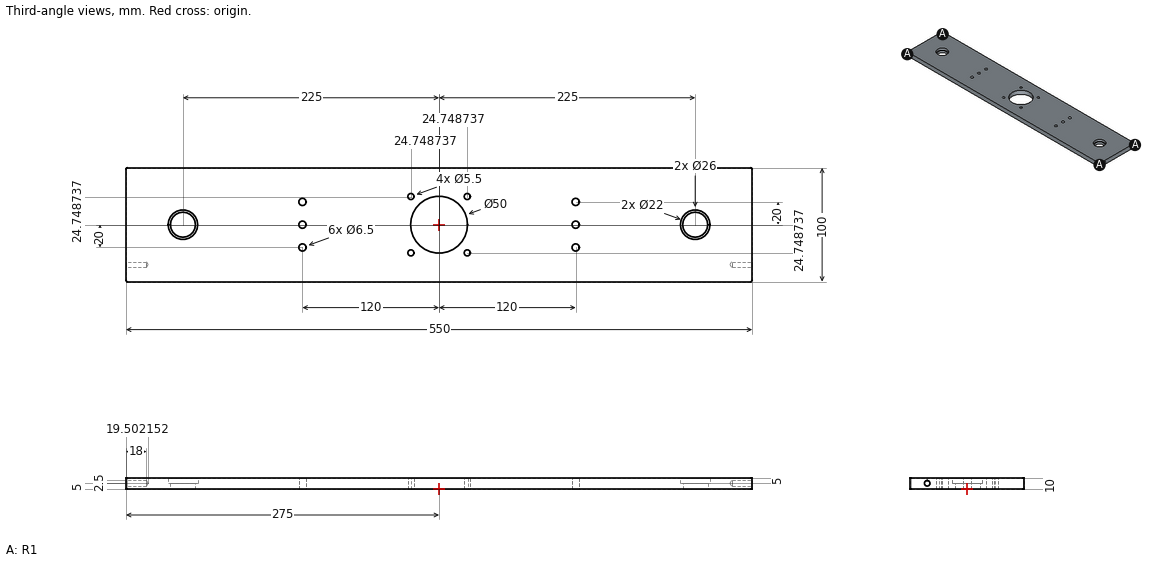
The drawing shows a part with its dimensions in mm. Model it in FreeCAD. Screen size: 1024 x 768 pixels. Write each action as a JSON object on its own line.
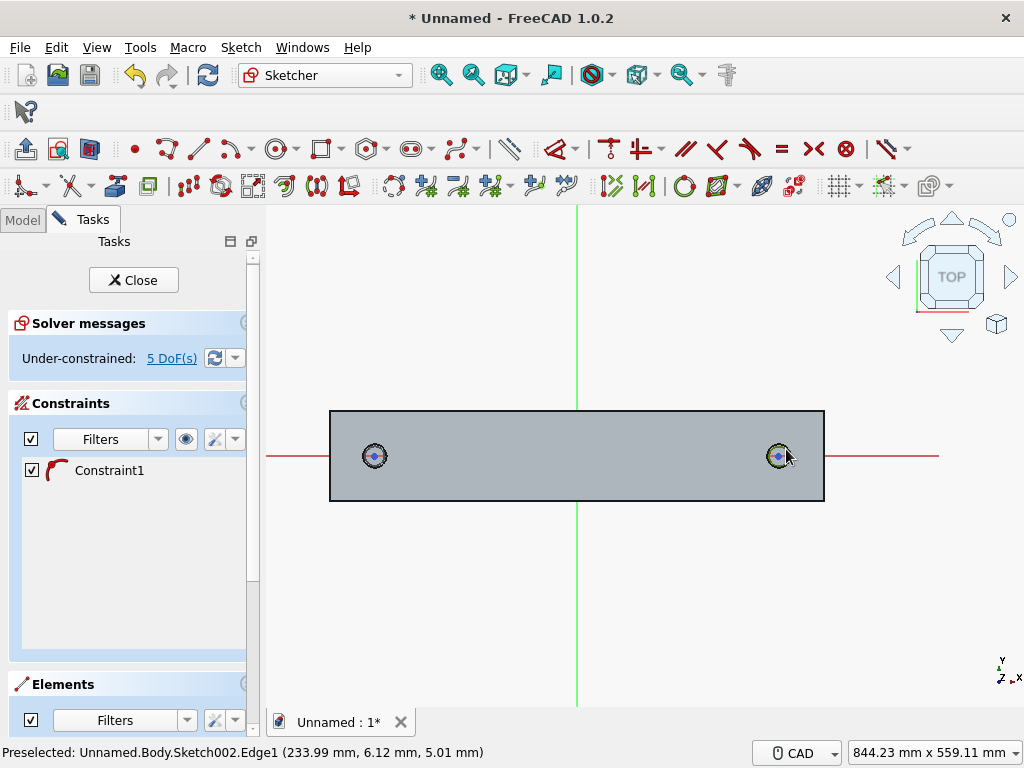
{"action": "scroll", "coordinate": [382, 449], "scroll_direction": "up", "scroll_amount": 4}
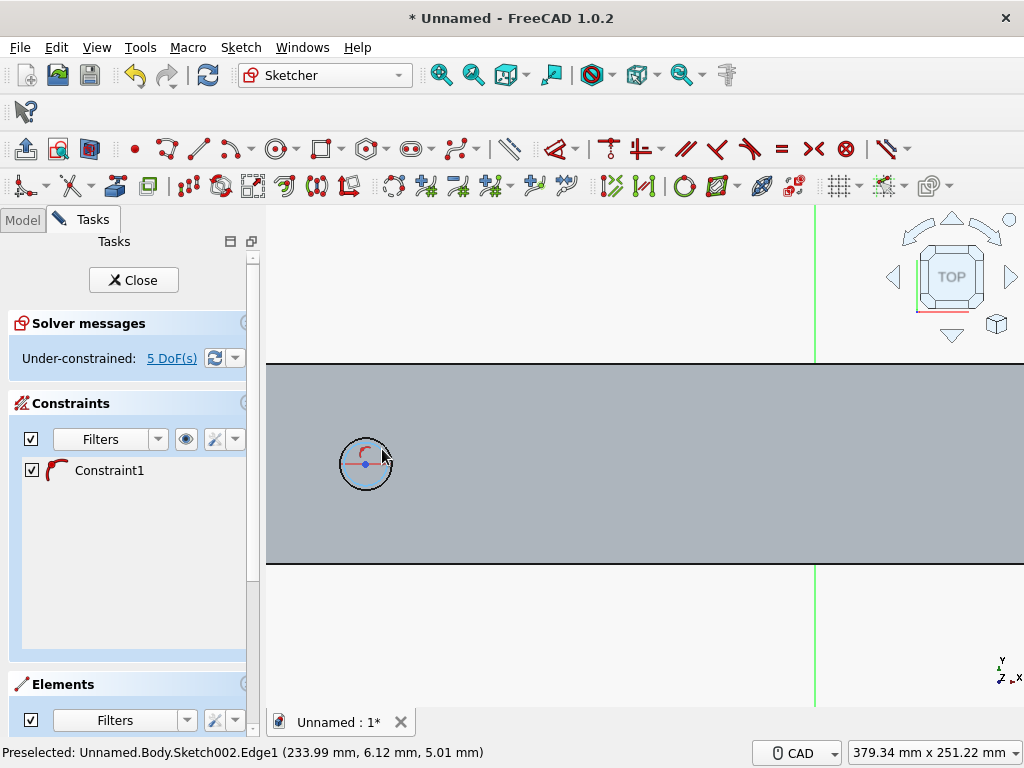
{"action": "left_click", "coordinate": [381, 449]}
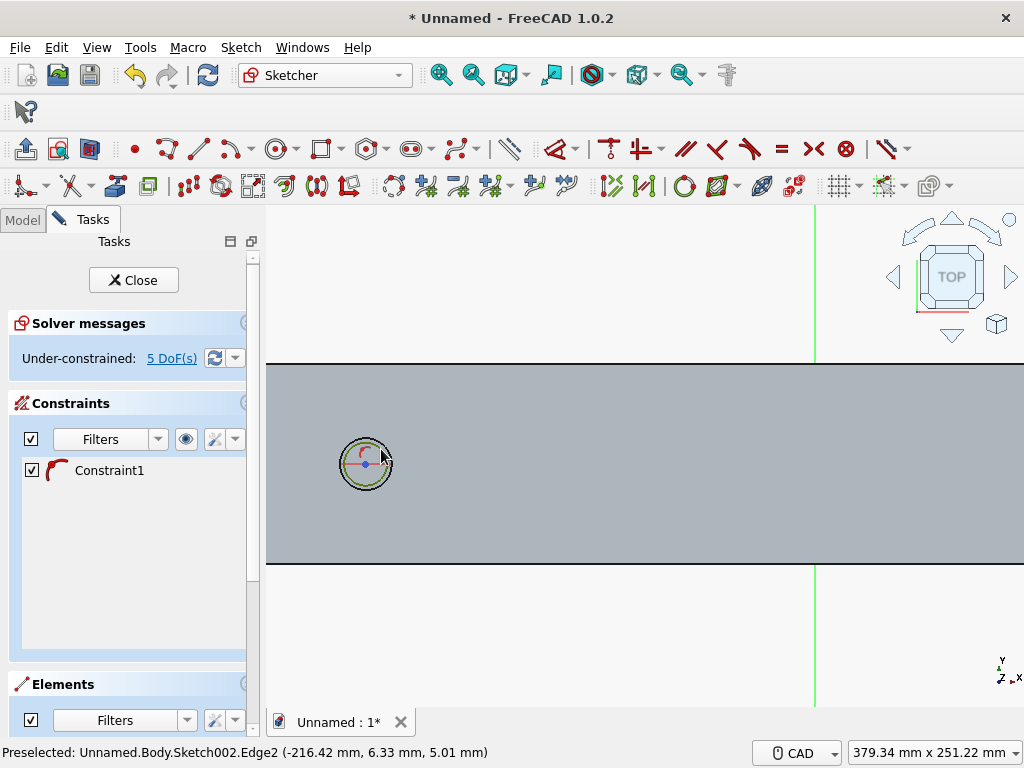
{"action": "left_click", "coordinate": [782, 150]}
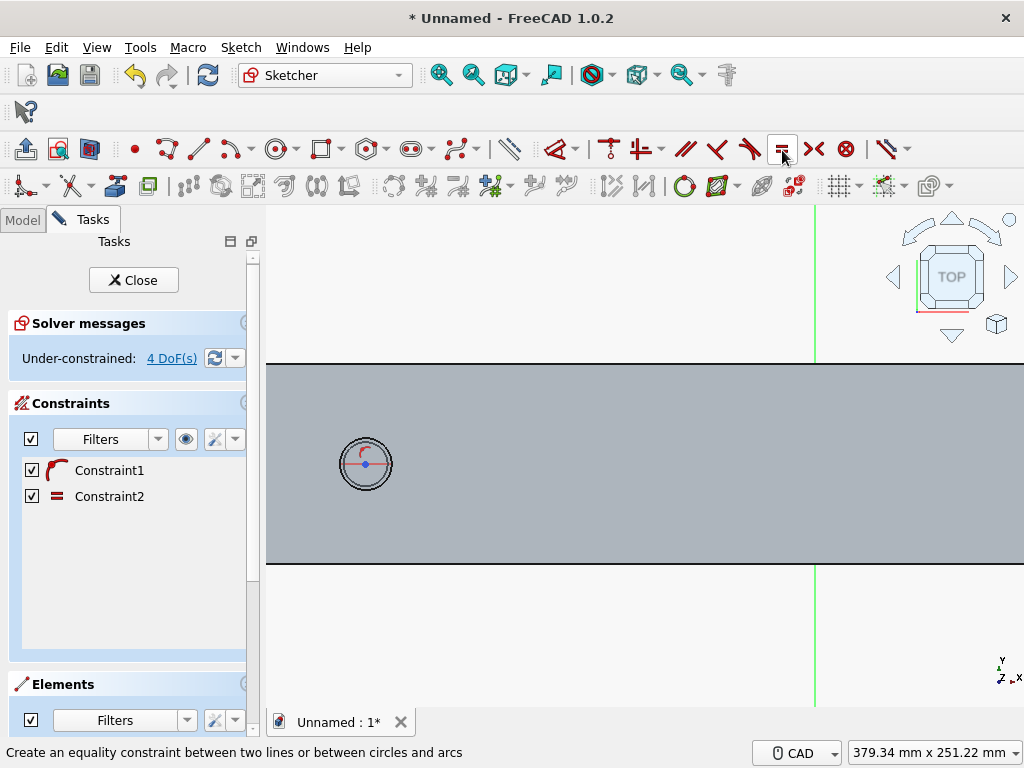
{"action": "scroll", "coordinate": [382, 449], "scroll_direction": "down", "scroll_amount": 4}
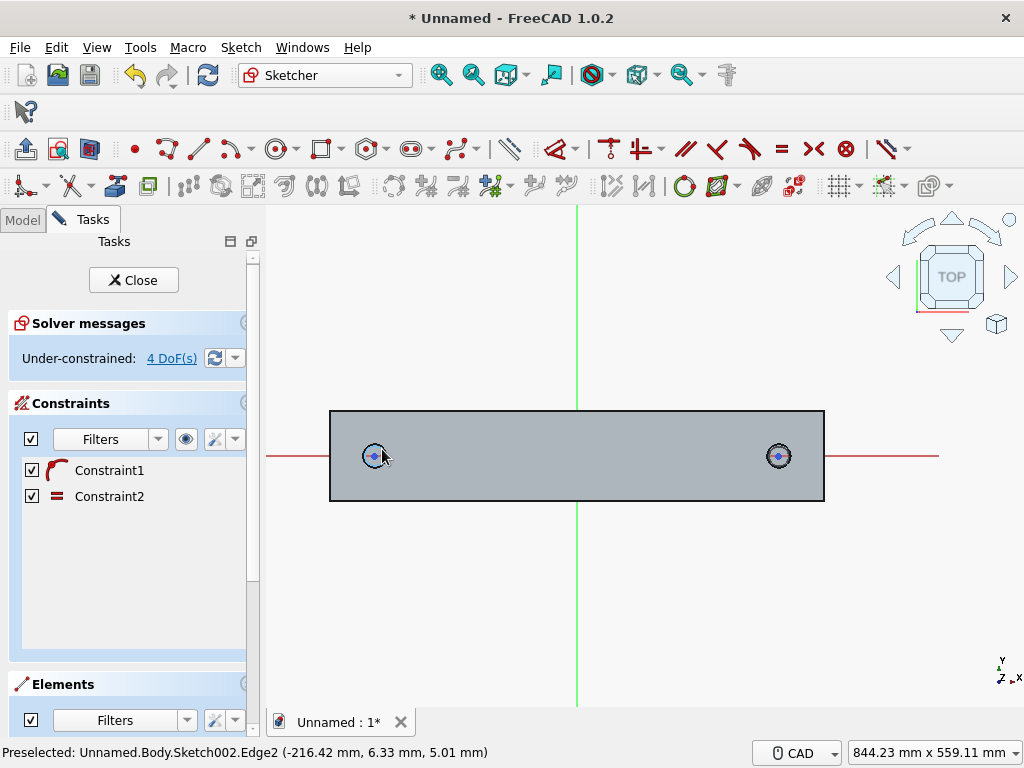
{"action": "left_click", "coordinate": [779, 456]}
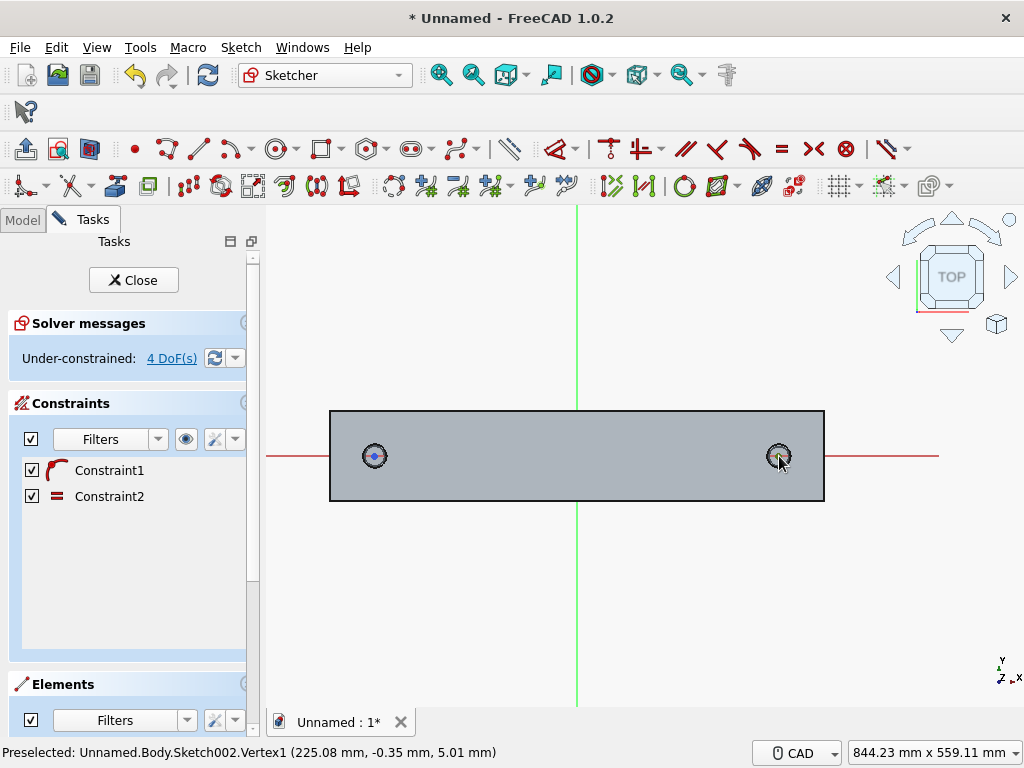
{"action": "left_click", "coordinate": [334, 456]}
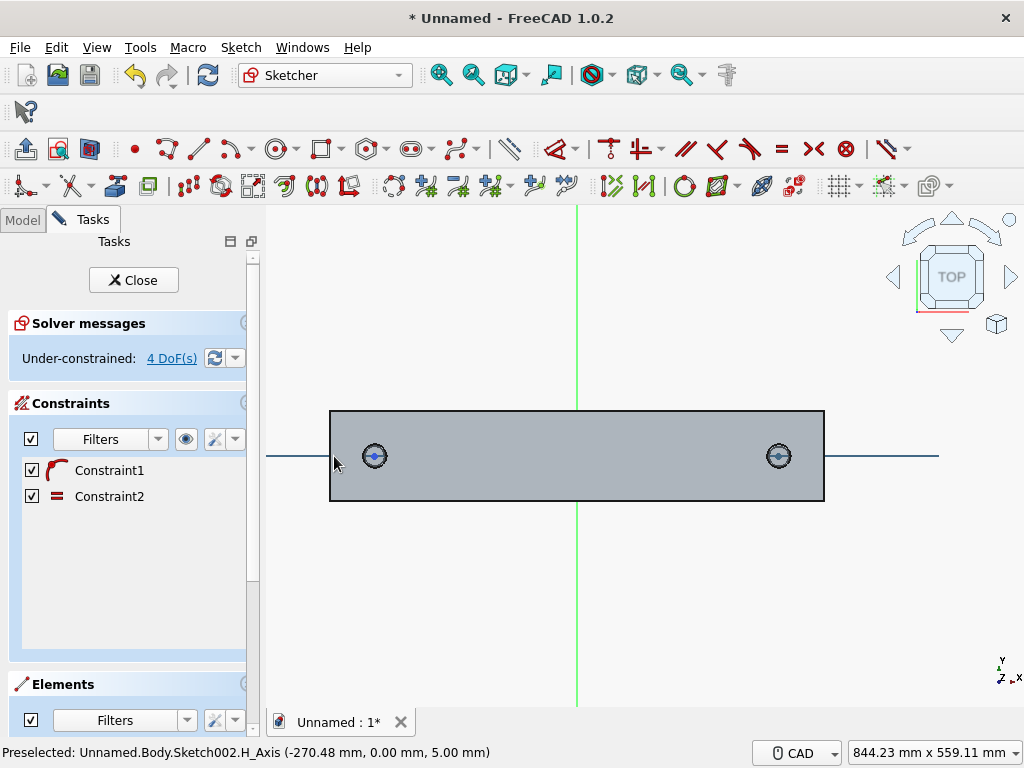
{"action": "key", "text": "c"}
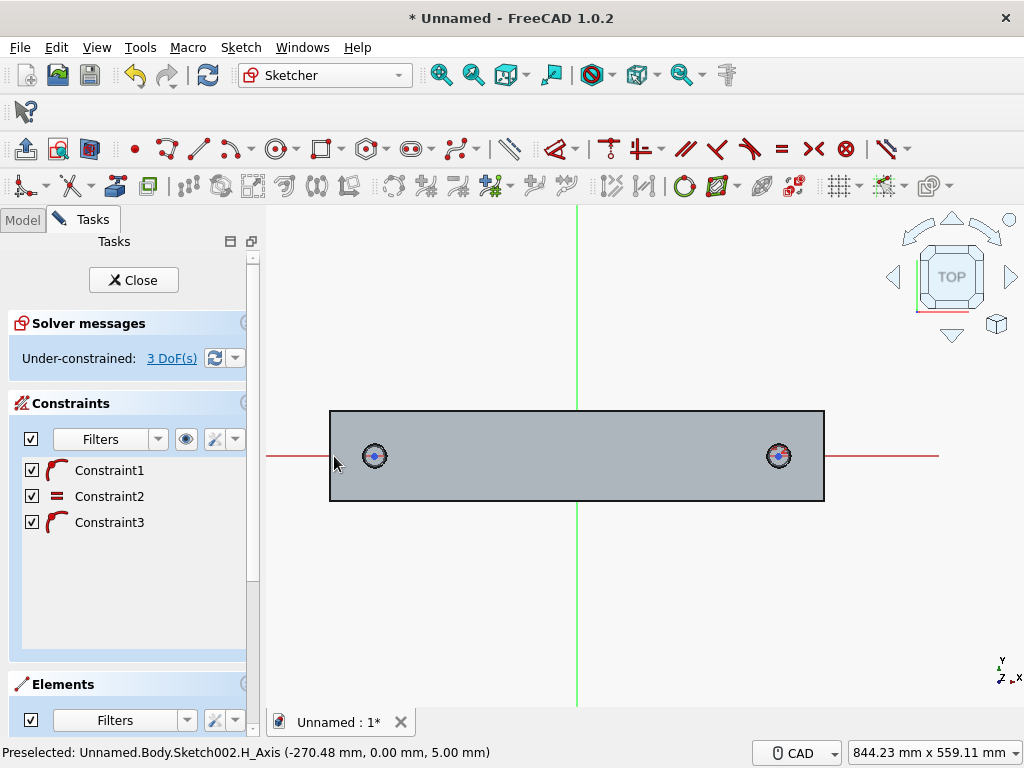
{"action": "key", "text": "d"}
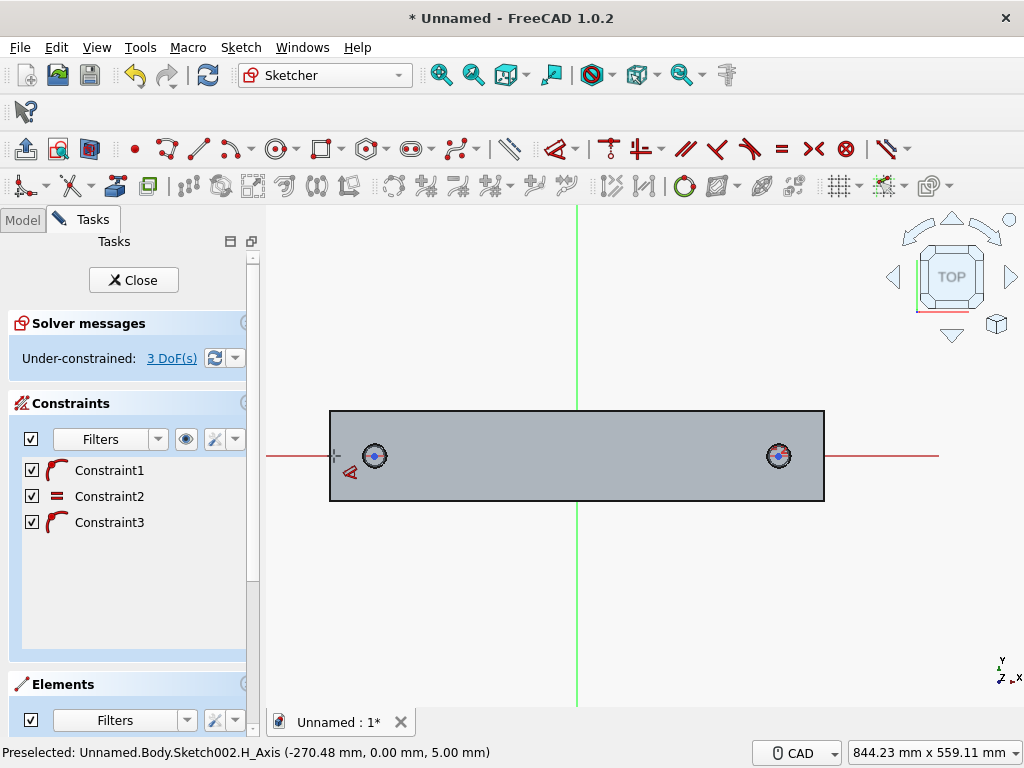
{"action": "scroll", "coordinate": [779, 446], "scroll_direction": "up", "scroll_amount": 4}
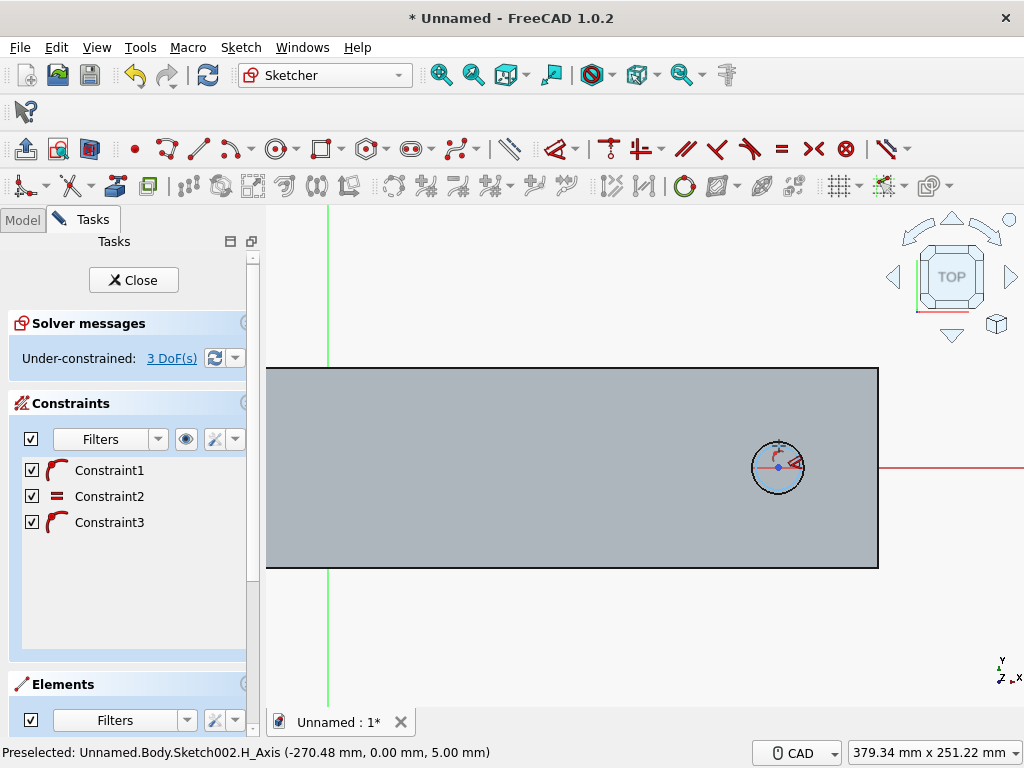
{"action": "left_click", "coordinate": [779, 446]}
{"action": "left_click", "coordinate": [780, 414]}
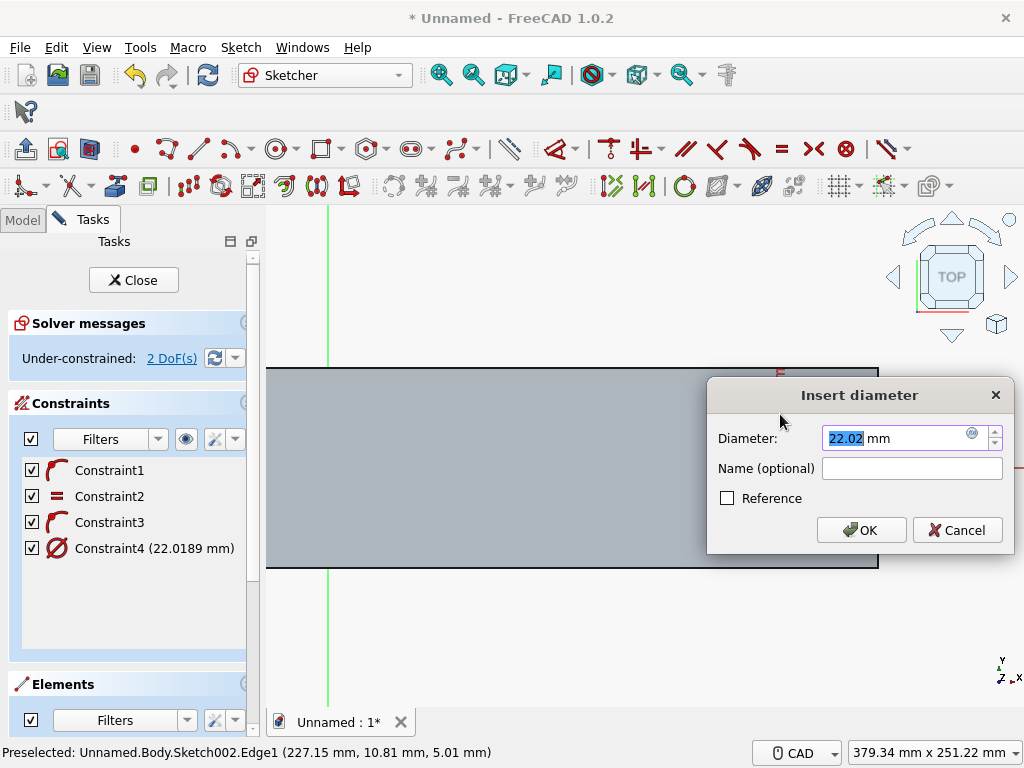
{"action": "type", "text": "22"}
{"action": "key", "text": "Return"}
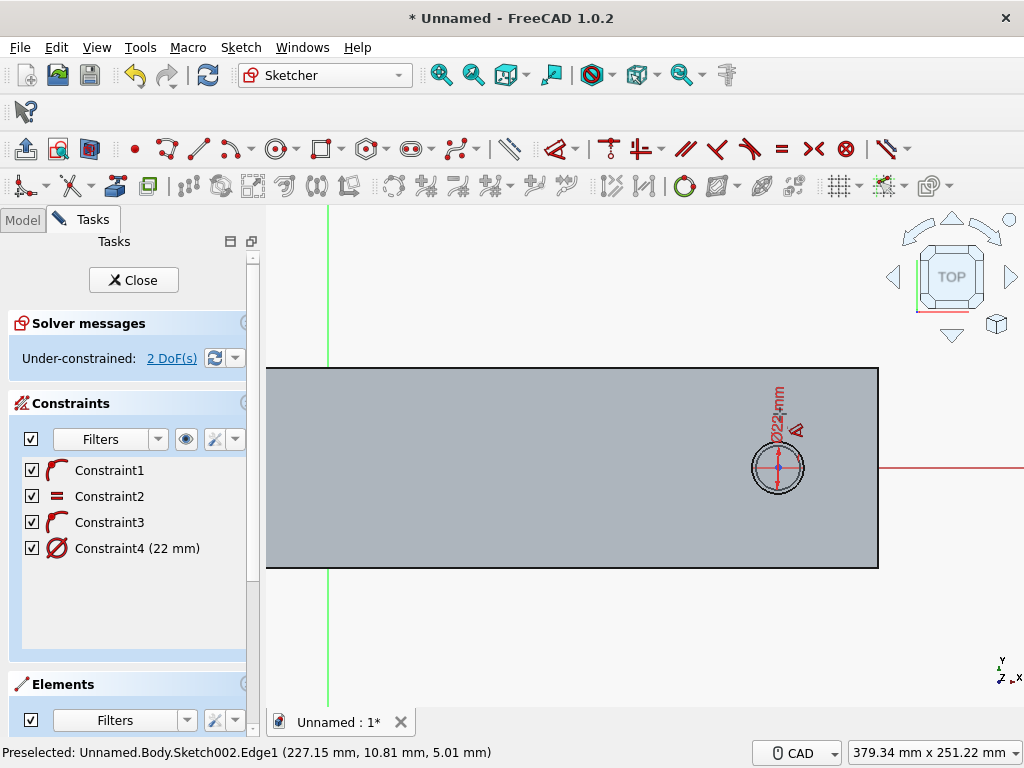
{"action": "left_click", "coordinate": [778, 468]}
{"action": "left_click", "coordinate": [553, 502]}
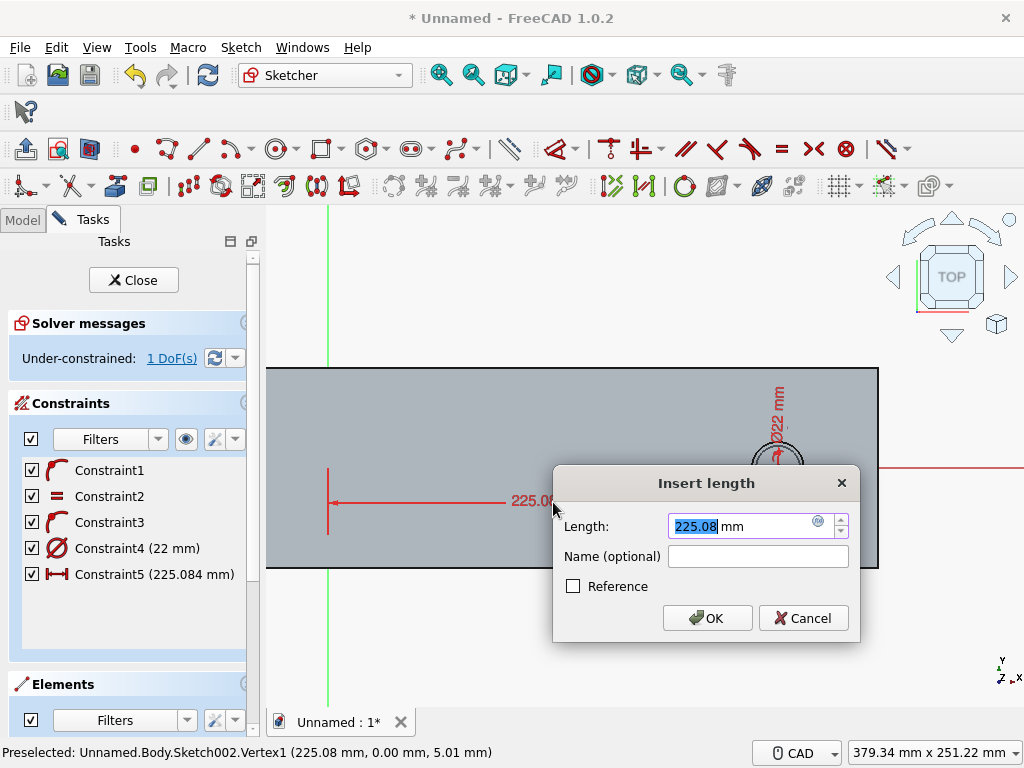
{"action": "type", "text": "225"}
{"action": "key", "text": "Return"}